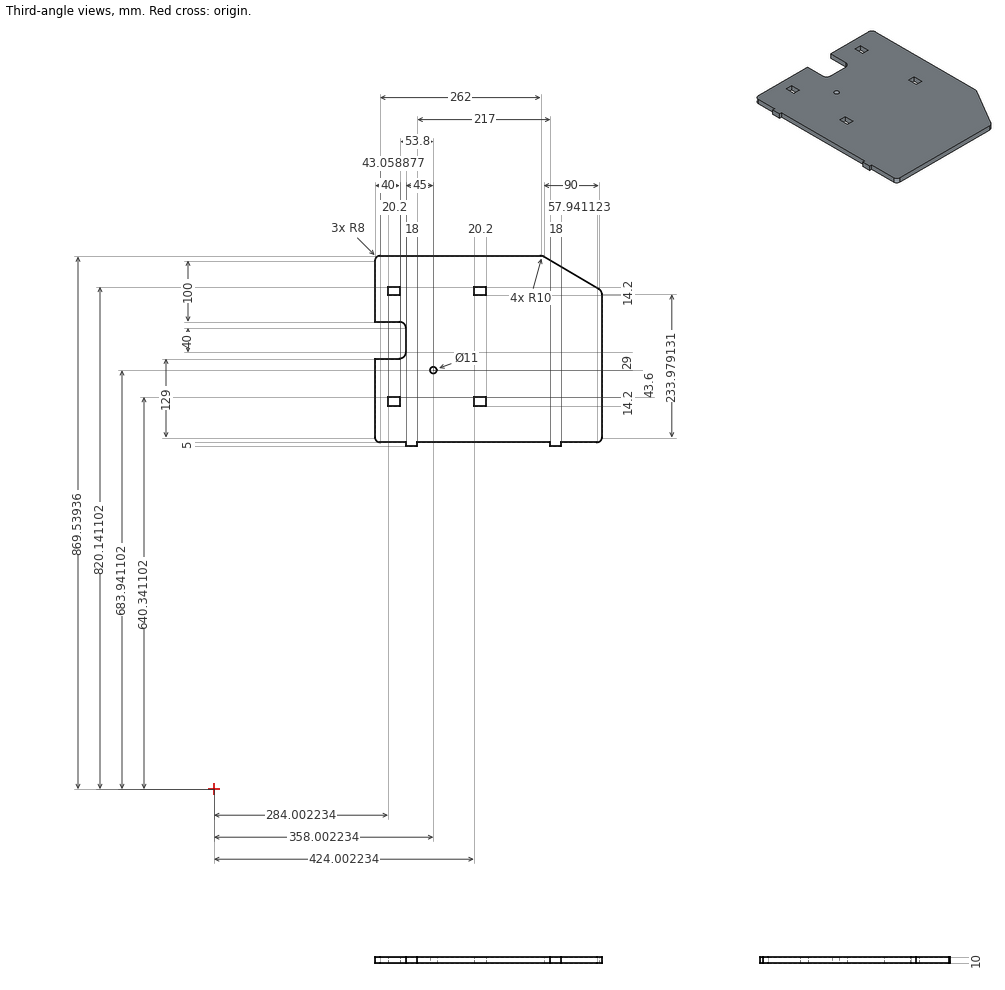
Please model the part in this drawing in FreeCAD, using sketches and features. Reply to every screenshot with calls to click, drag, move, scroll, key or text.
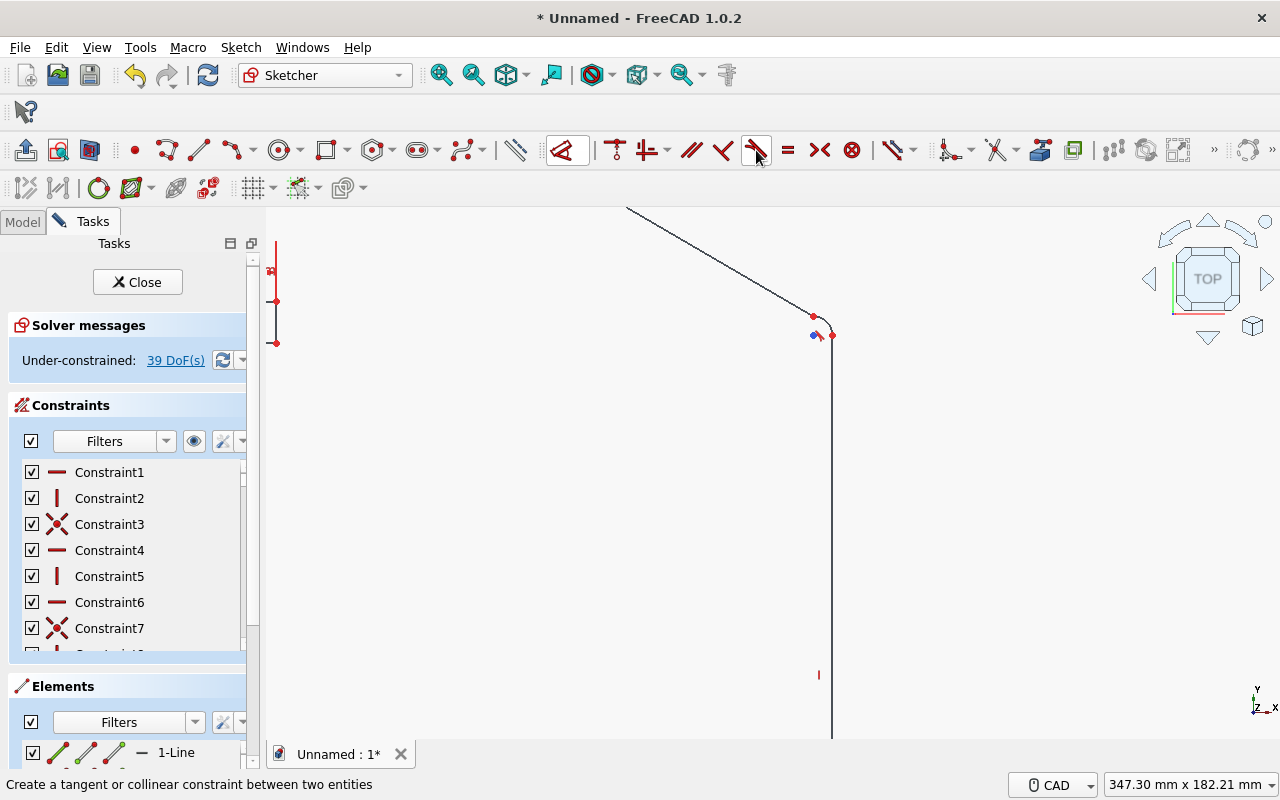
scroll(830, 324, down, 10)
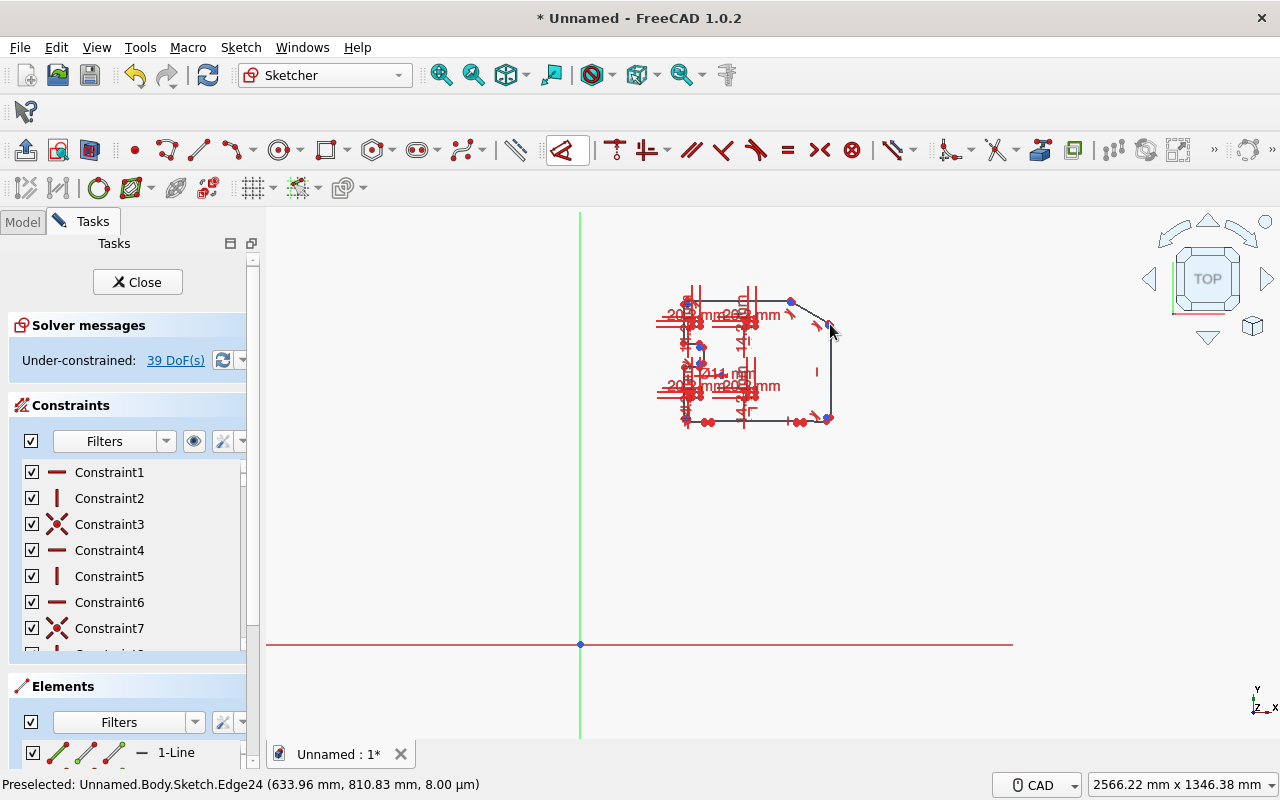
scroll(799, 423, up, 10)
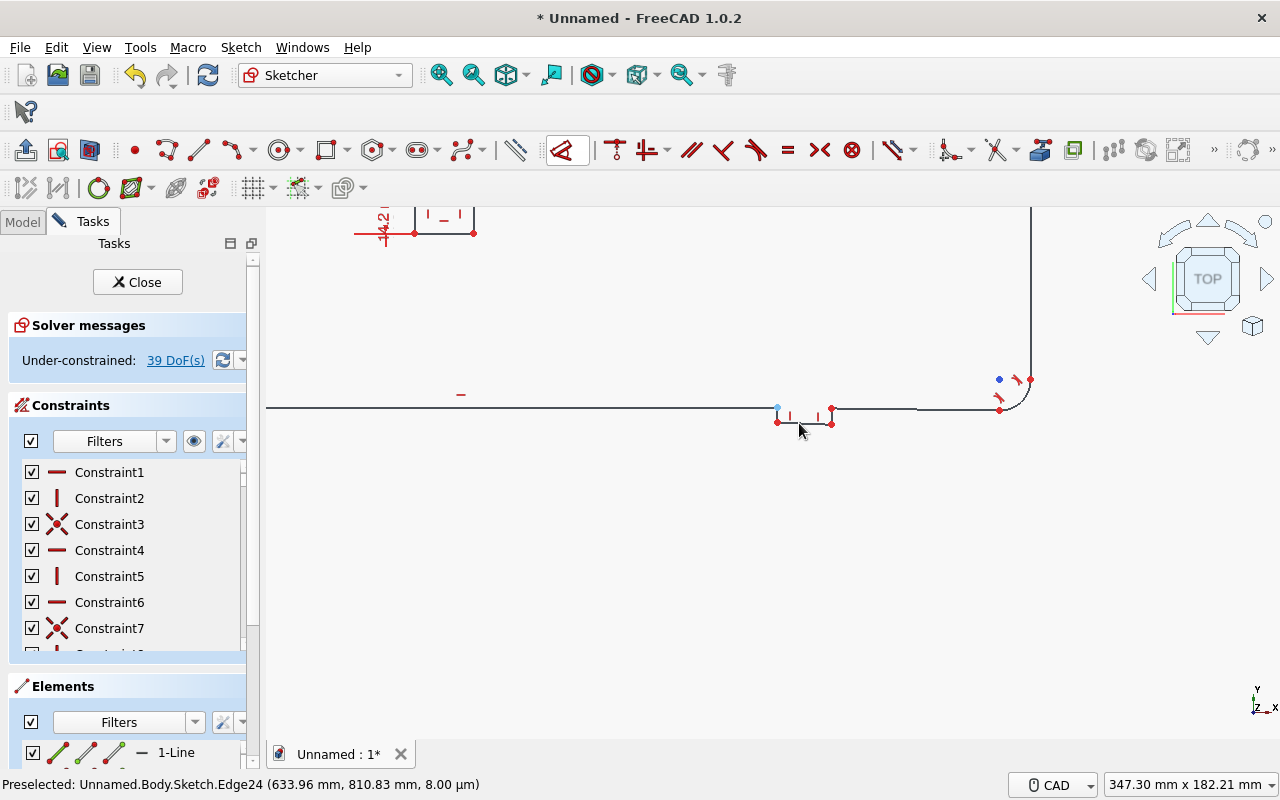
click(794, 423)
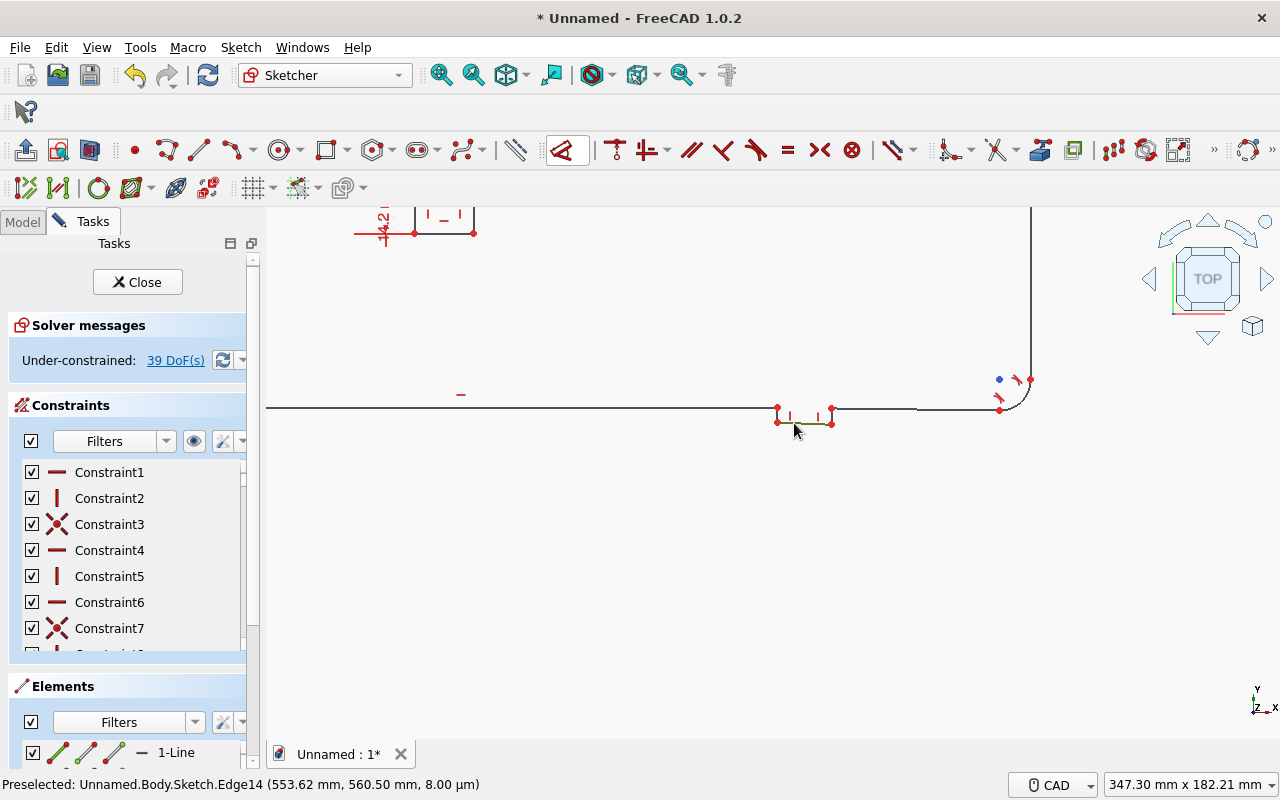
click(670, 150)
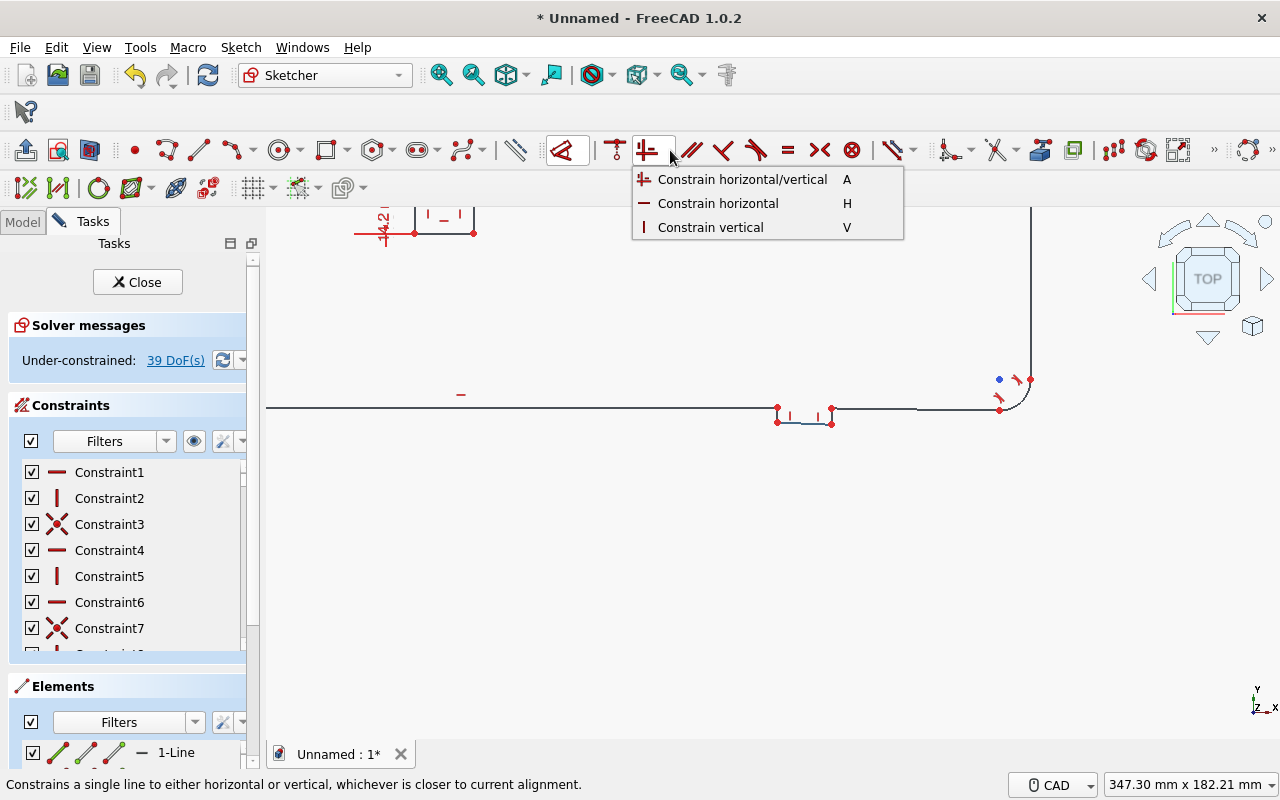
click(768, 203)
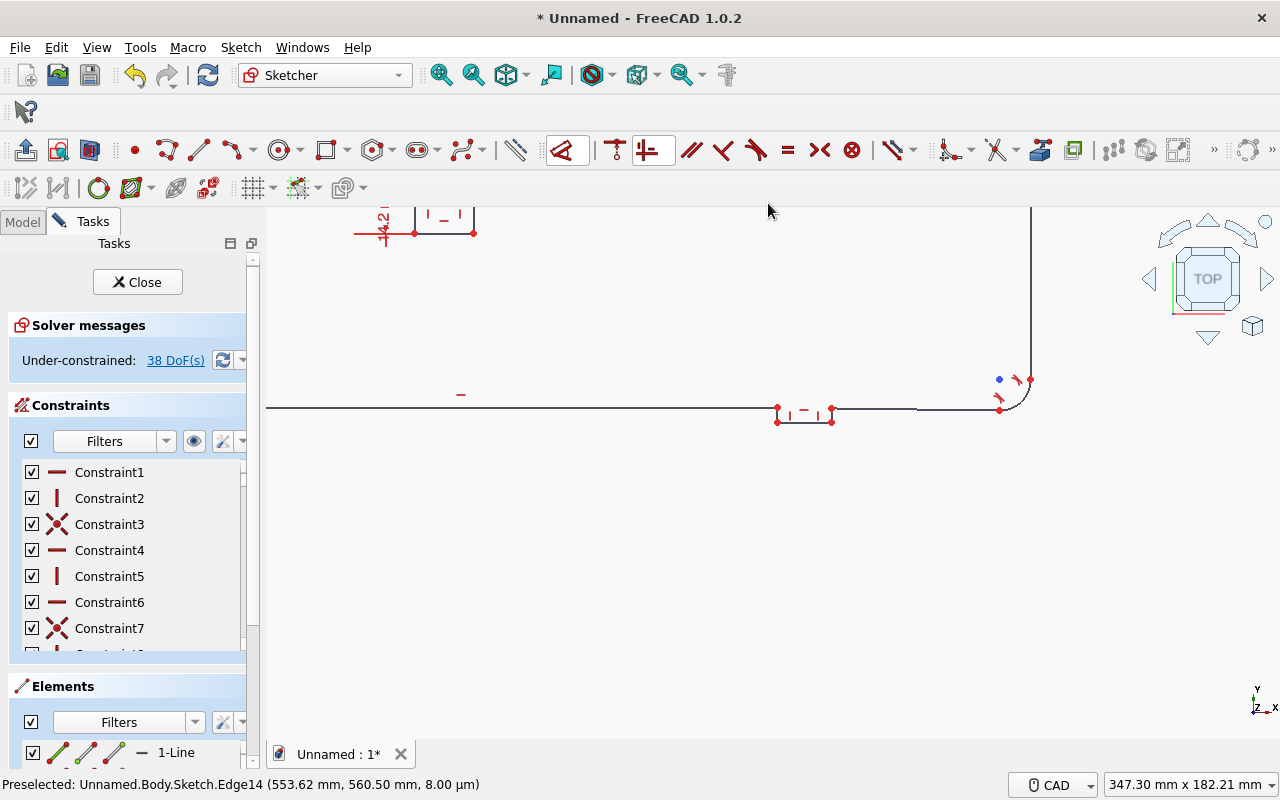
scroll(799, 424, down, 10)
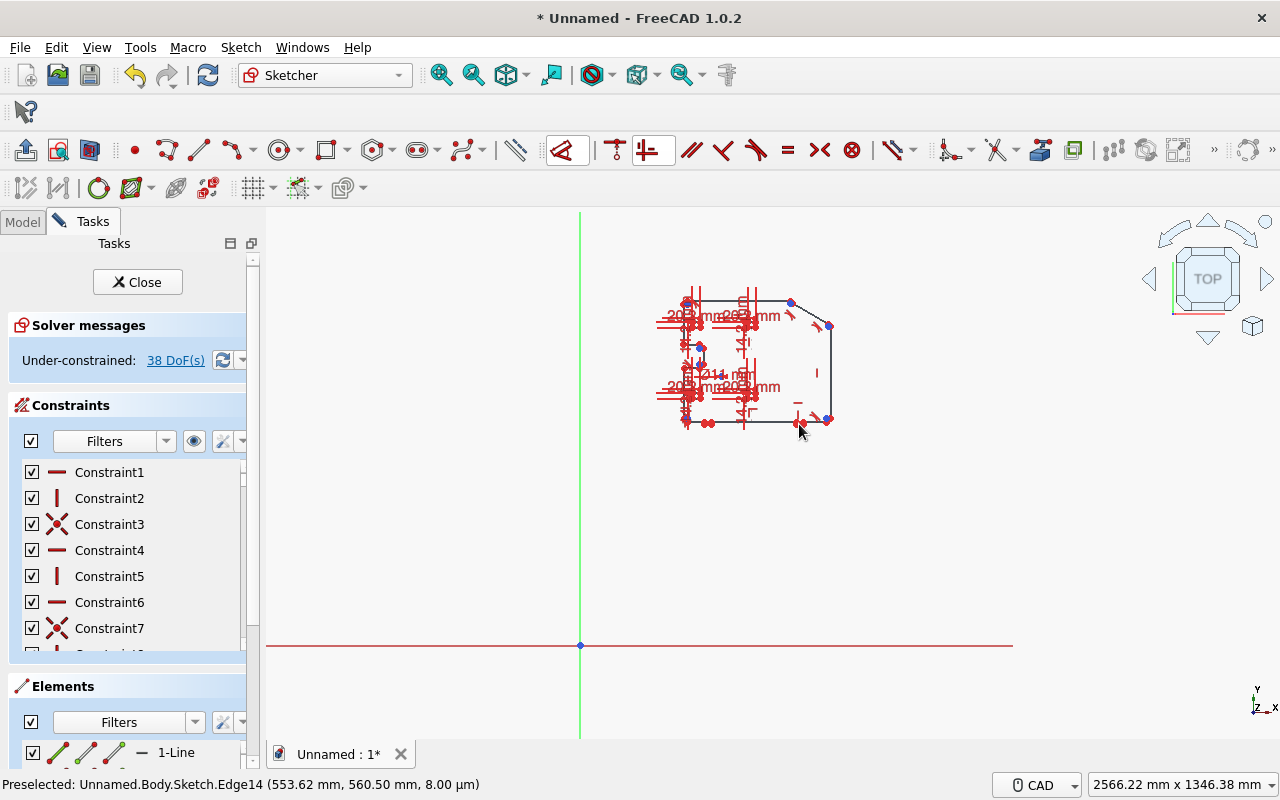
scroll(811, 422, up, 4)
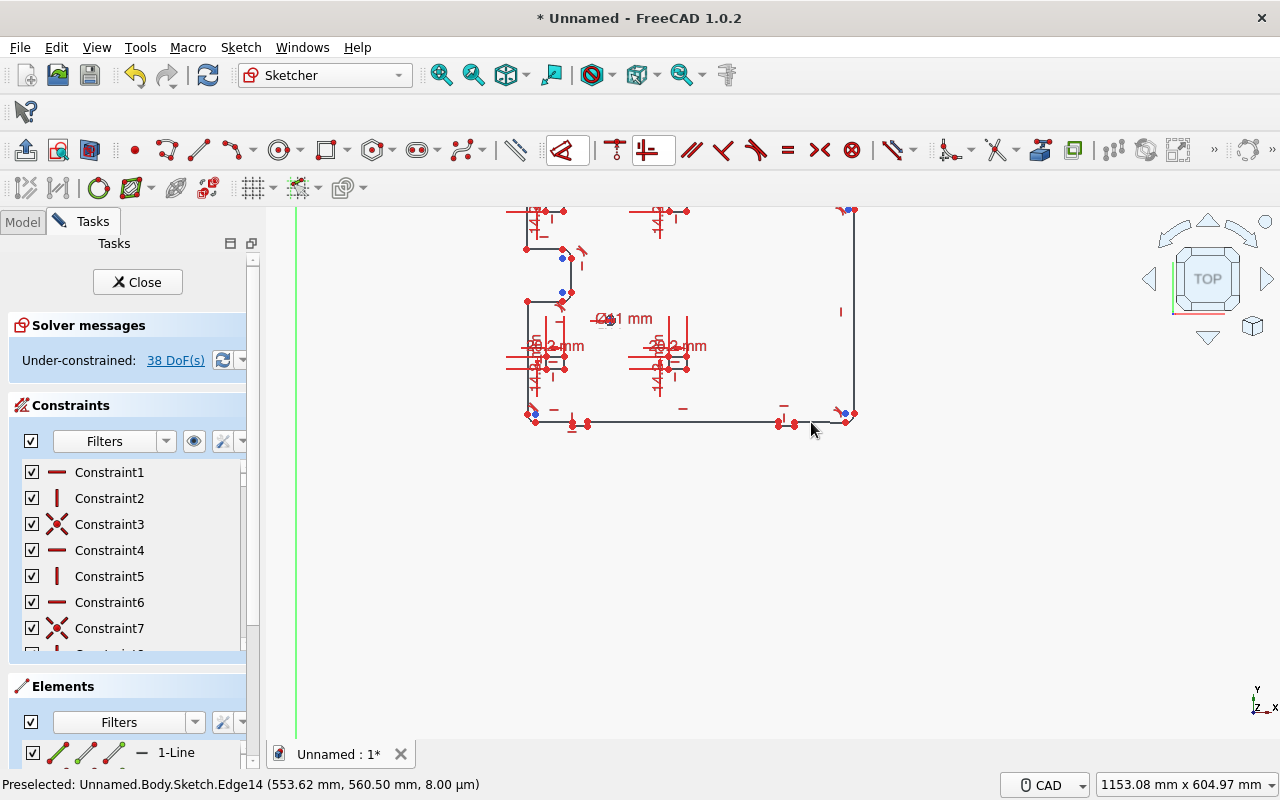
click(810, 422)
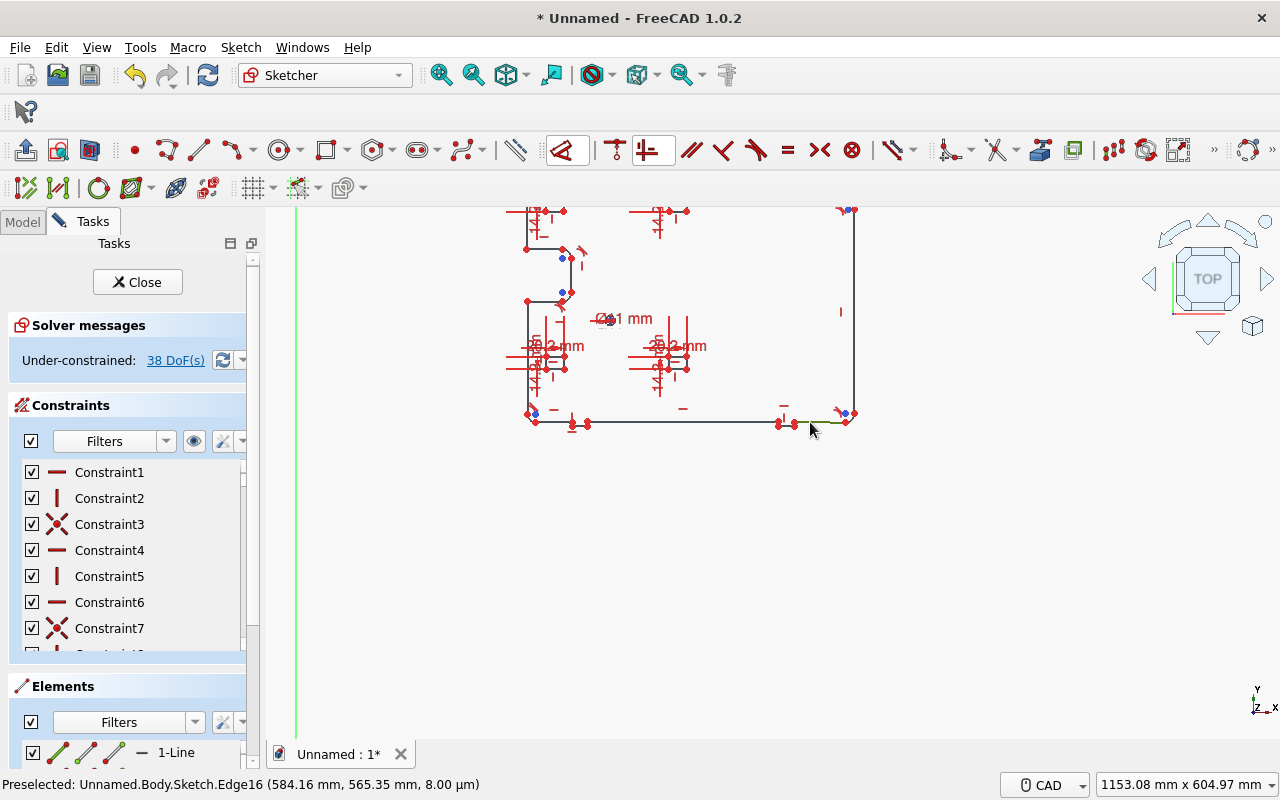
click(670, 150)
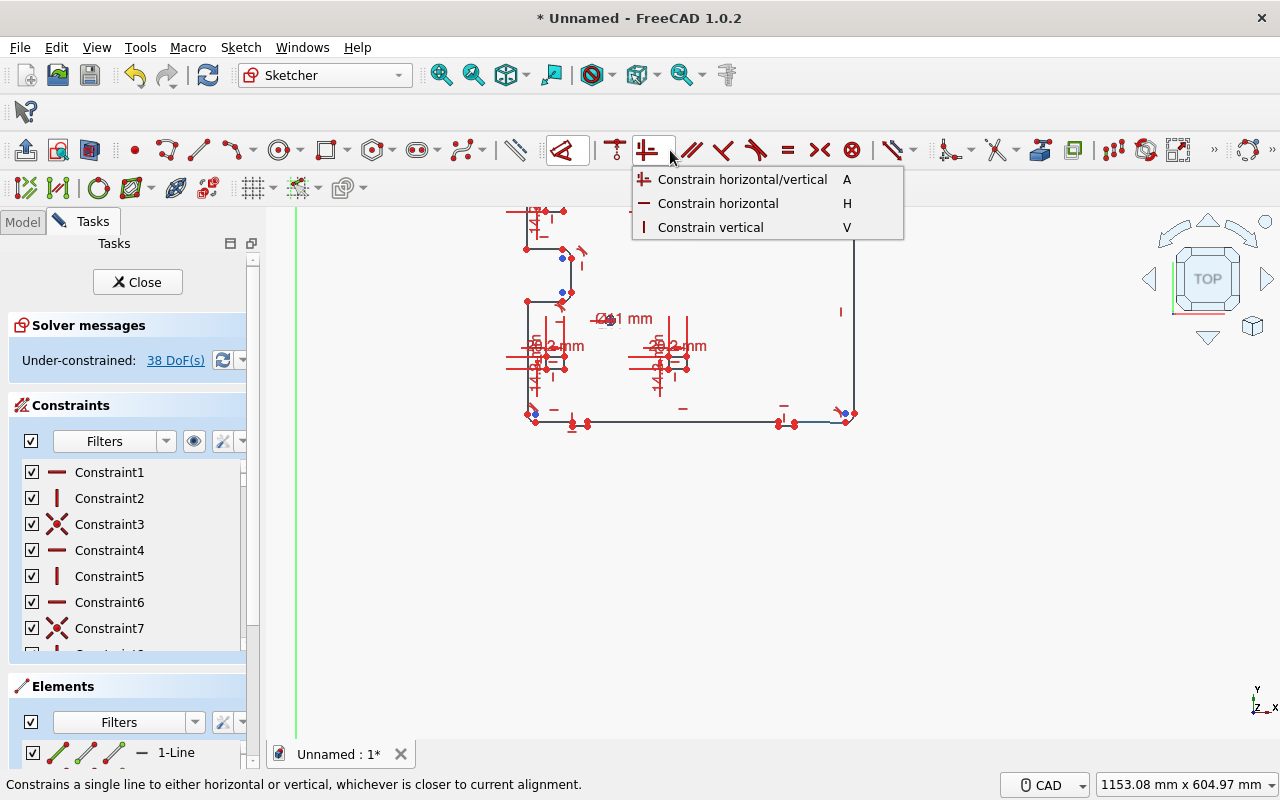
click(768, 203)